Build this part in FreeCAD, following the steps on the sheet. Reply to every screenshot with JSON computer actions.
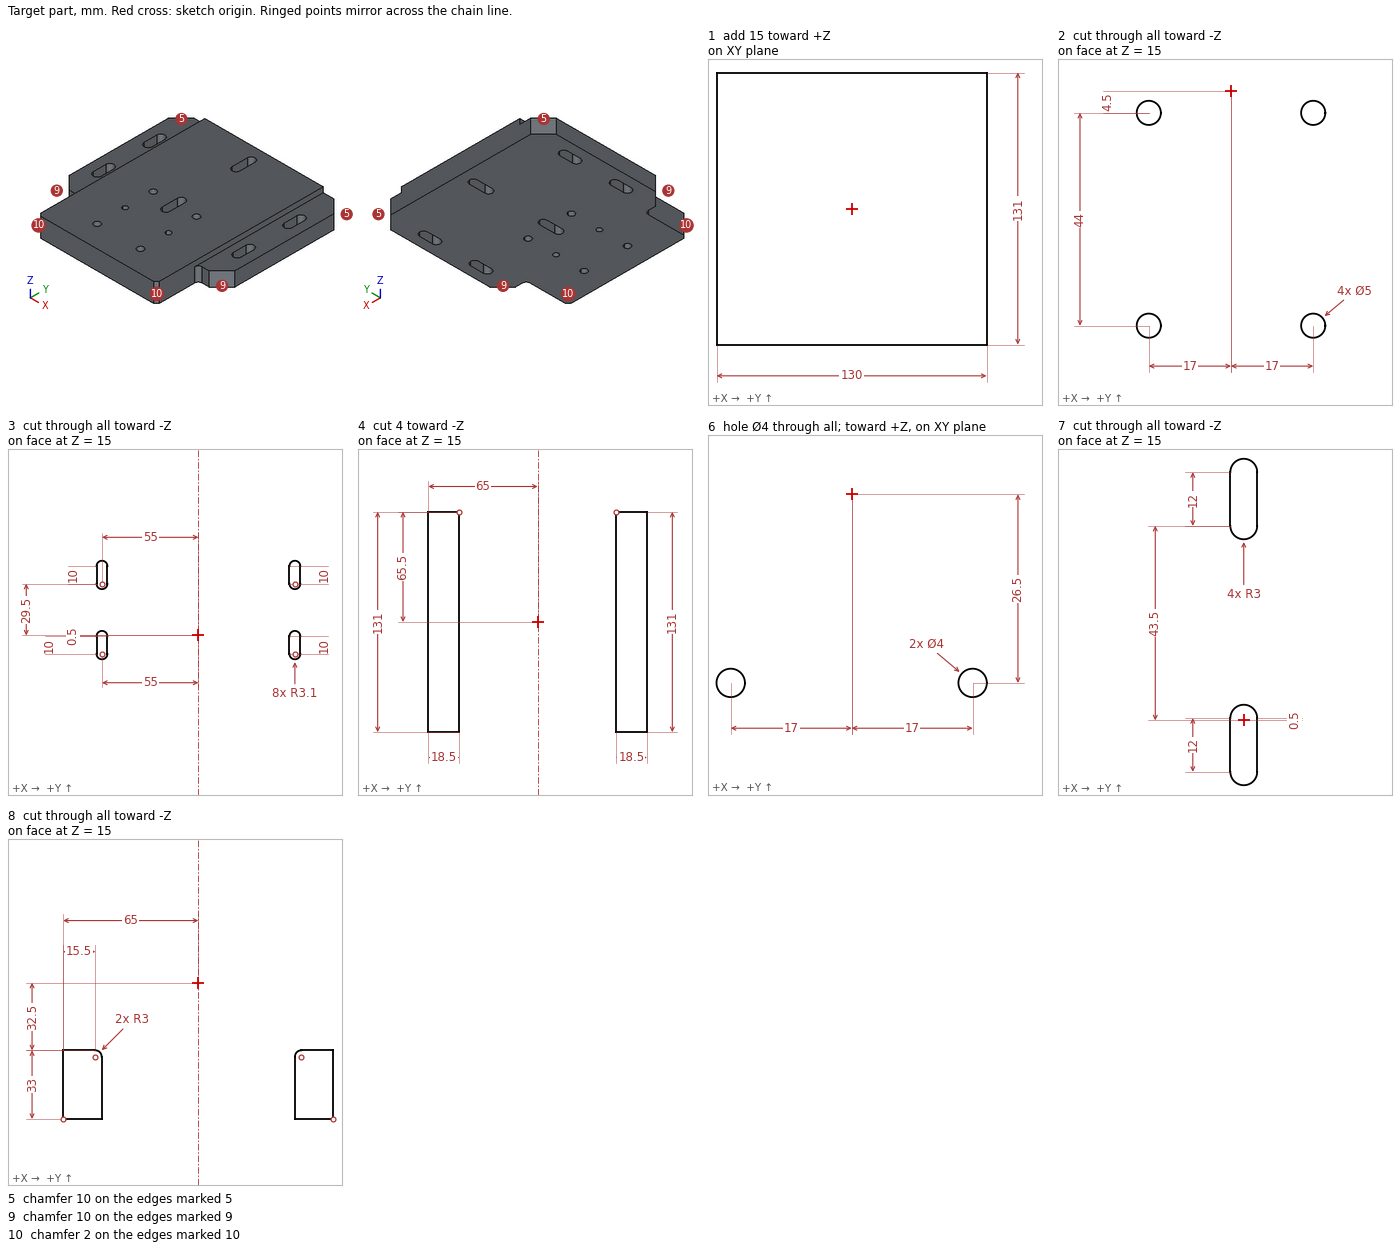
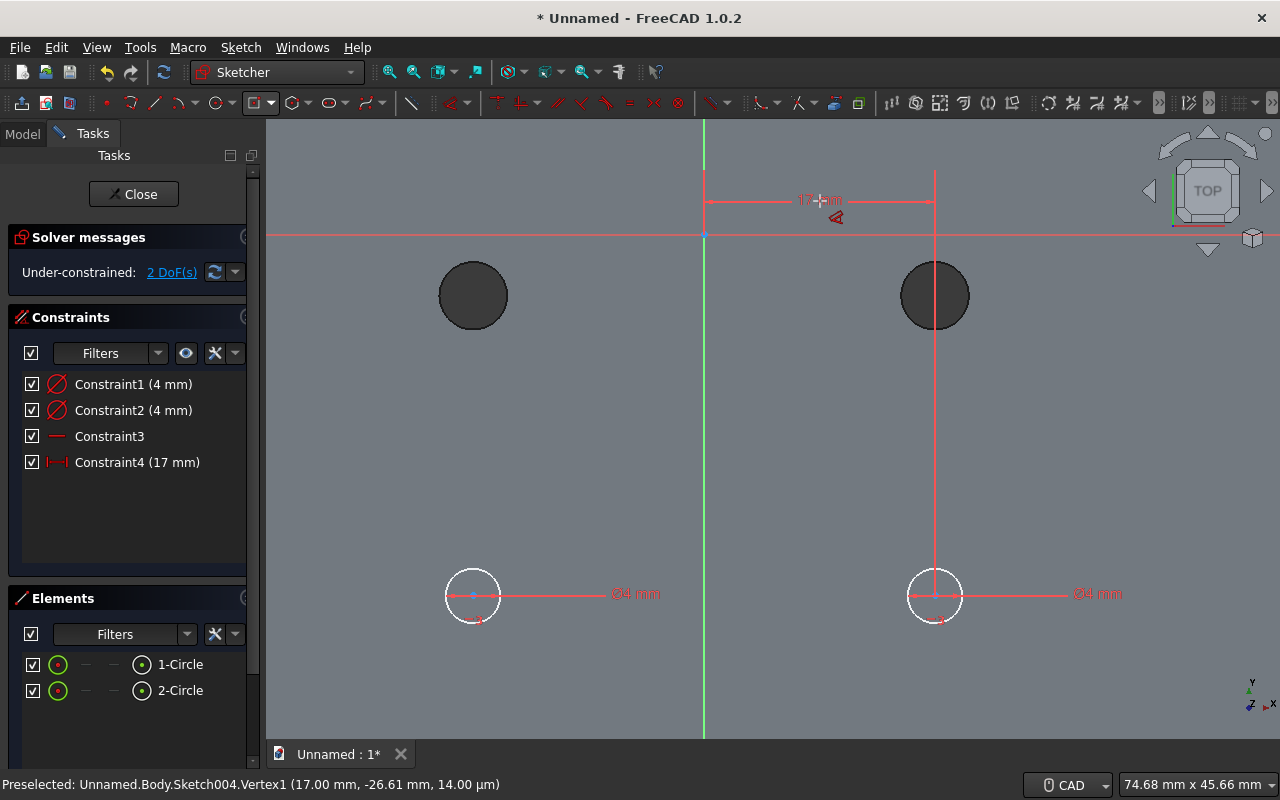
{"action": "left_click", "coordinate": [473, 596]}
{"action": "left_click", "coordinate": [589, 201]}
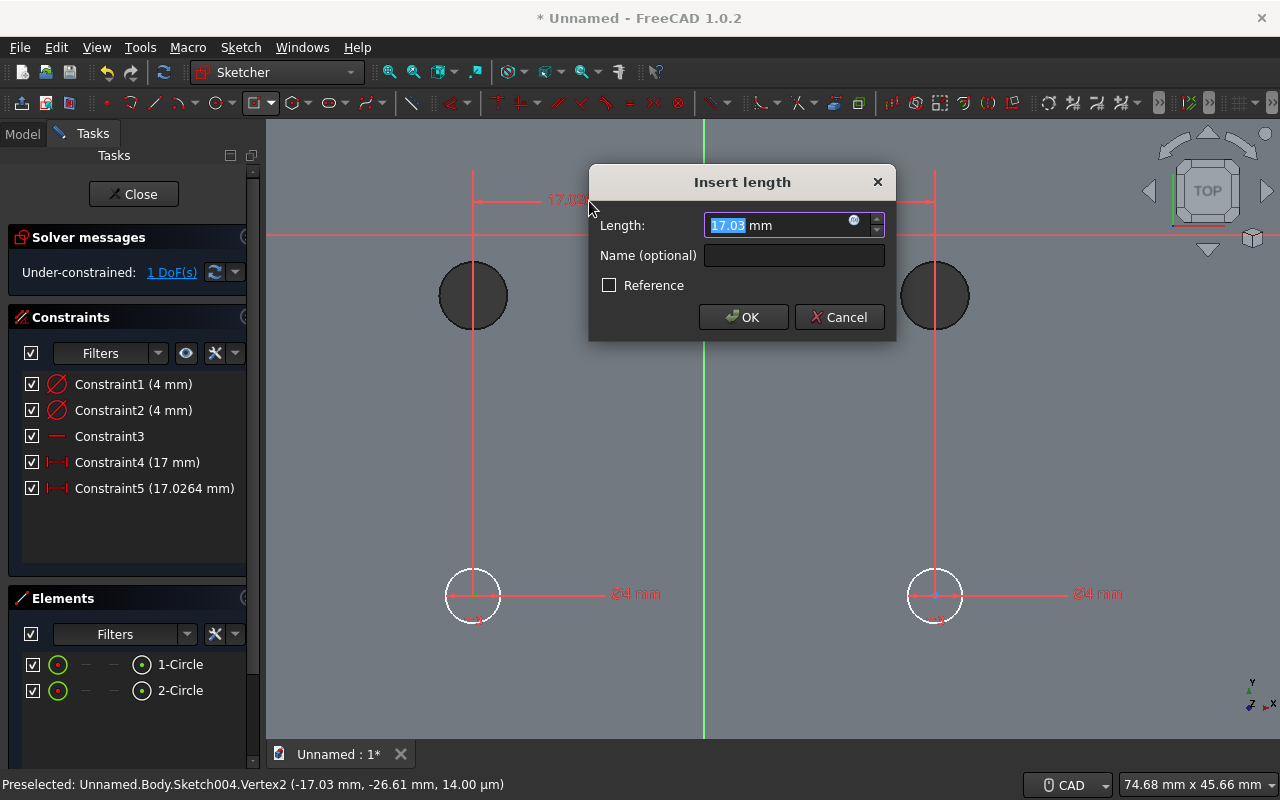
{"action": "type", "text": "17"}
{"action": "key", "text": "Return"}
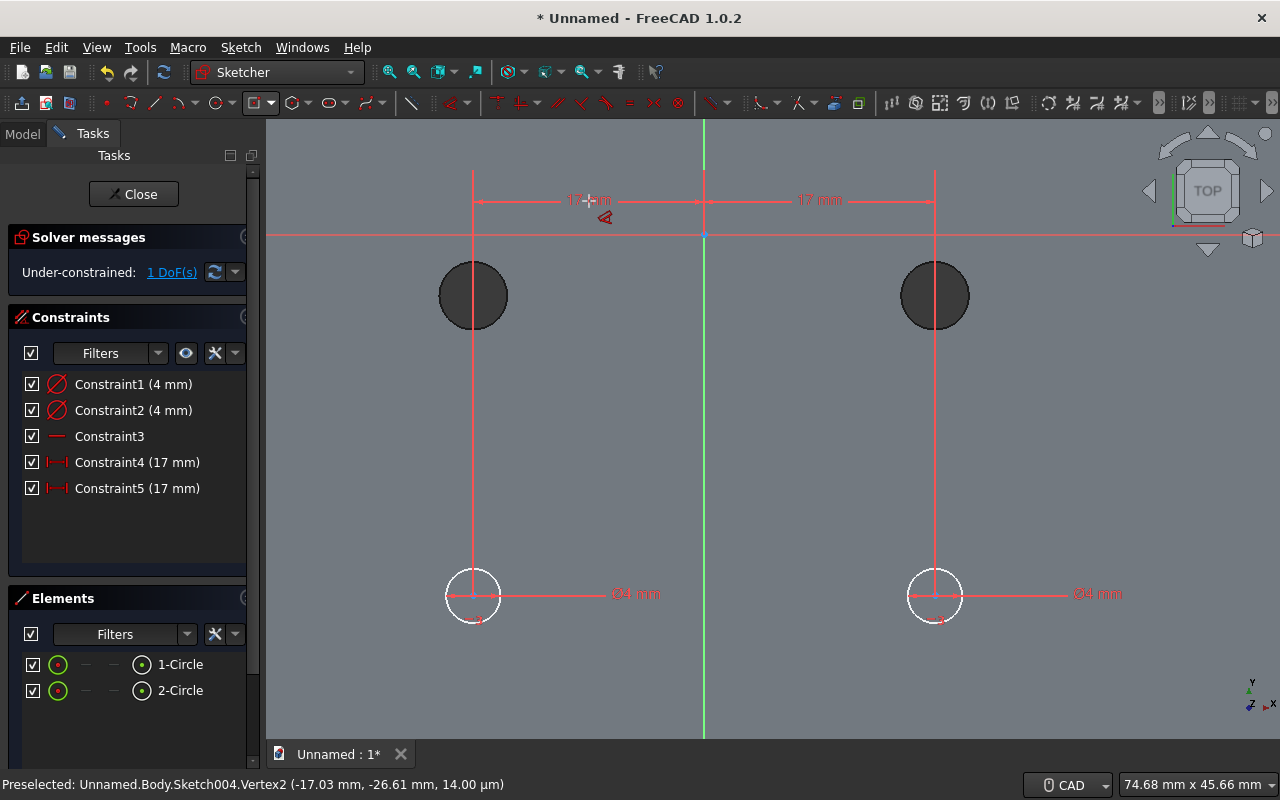
{"action": "left_click", "coordinate": [935, 596]}
{"action": "left_click", "coordinate": [969, 415]}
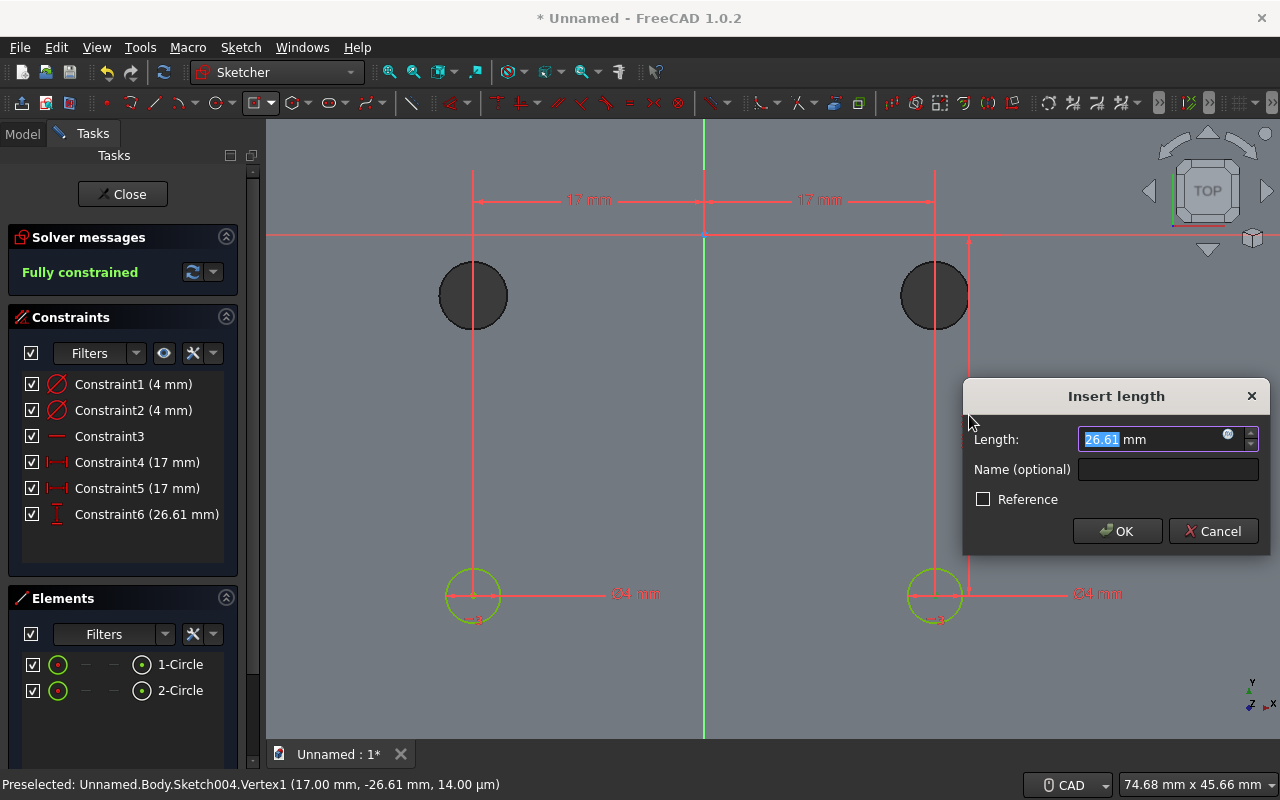
{"action": "type", "text": "26.5"}
{"action": "key", "text": "Return"}
{"action": "key", "text": "Escape"}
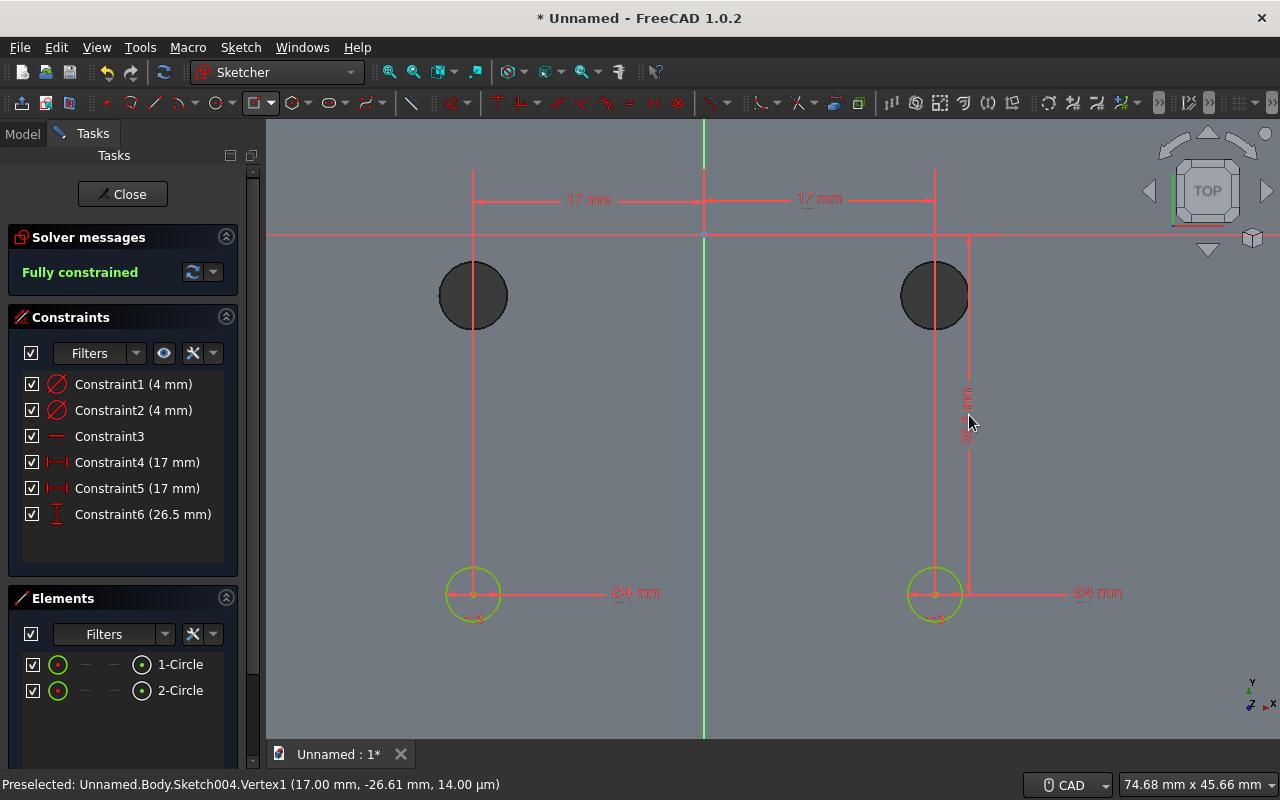
{"action": "left_click", "coordinate": [123, 194]}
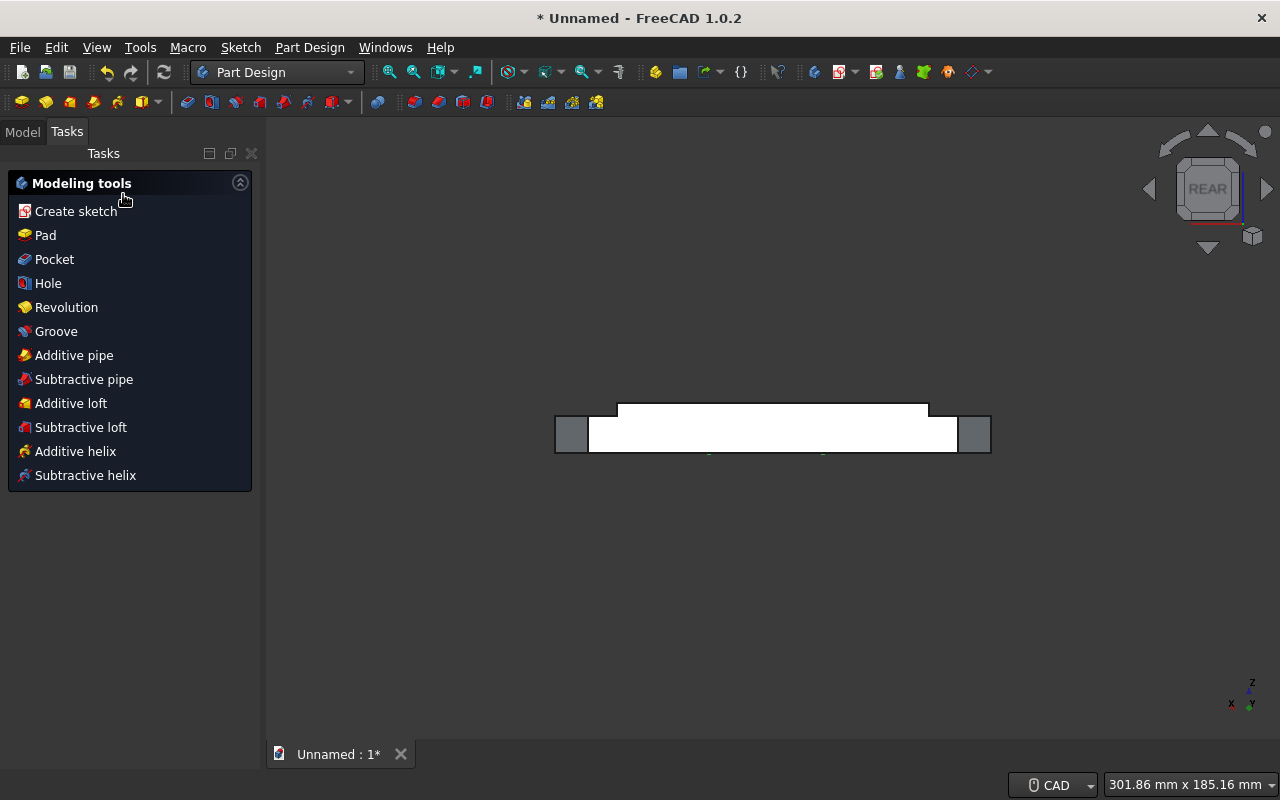
{"action": "left_click", "coordinate": [212, 102]}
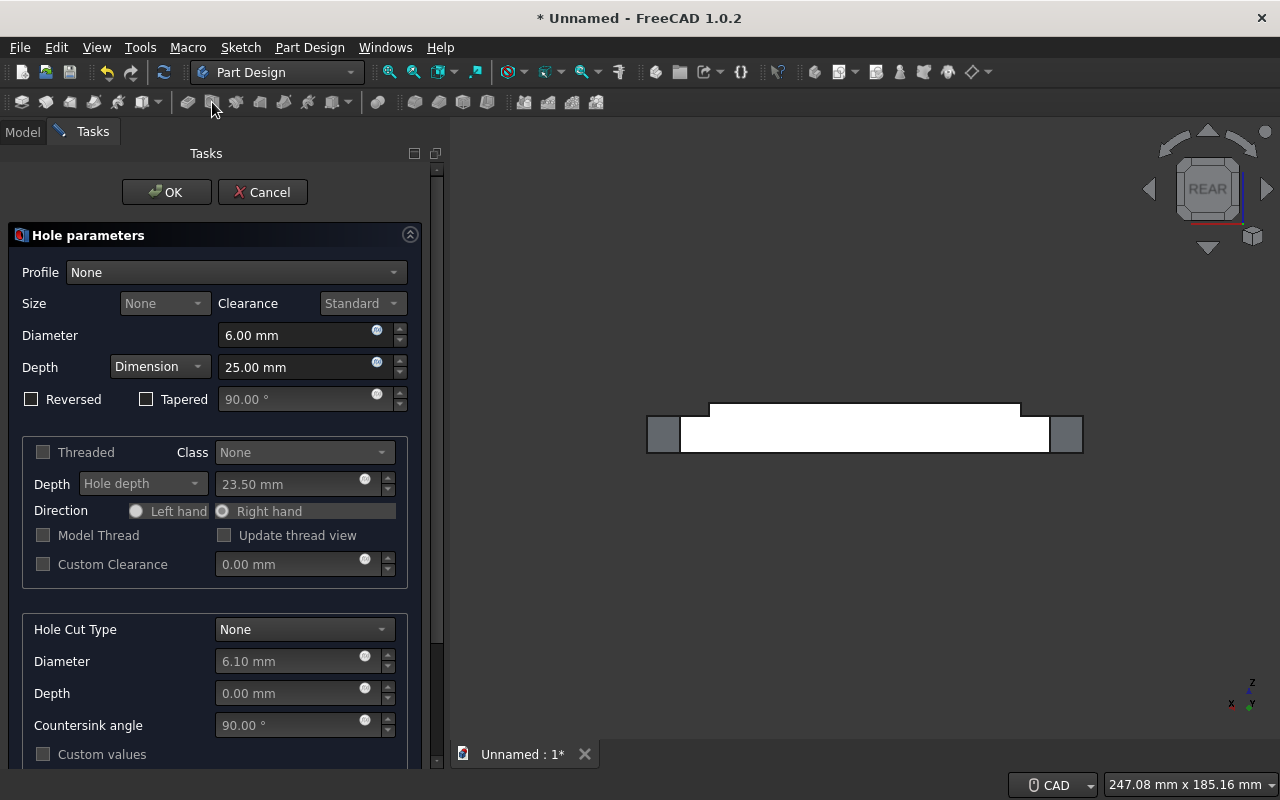
{"action": "triple_click", "coordinate": [305, 335]}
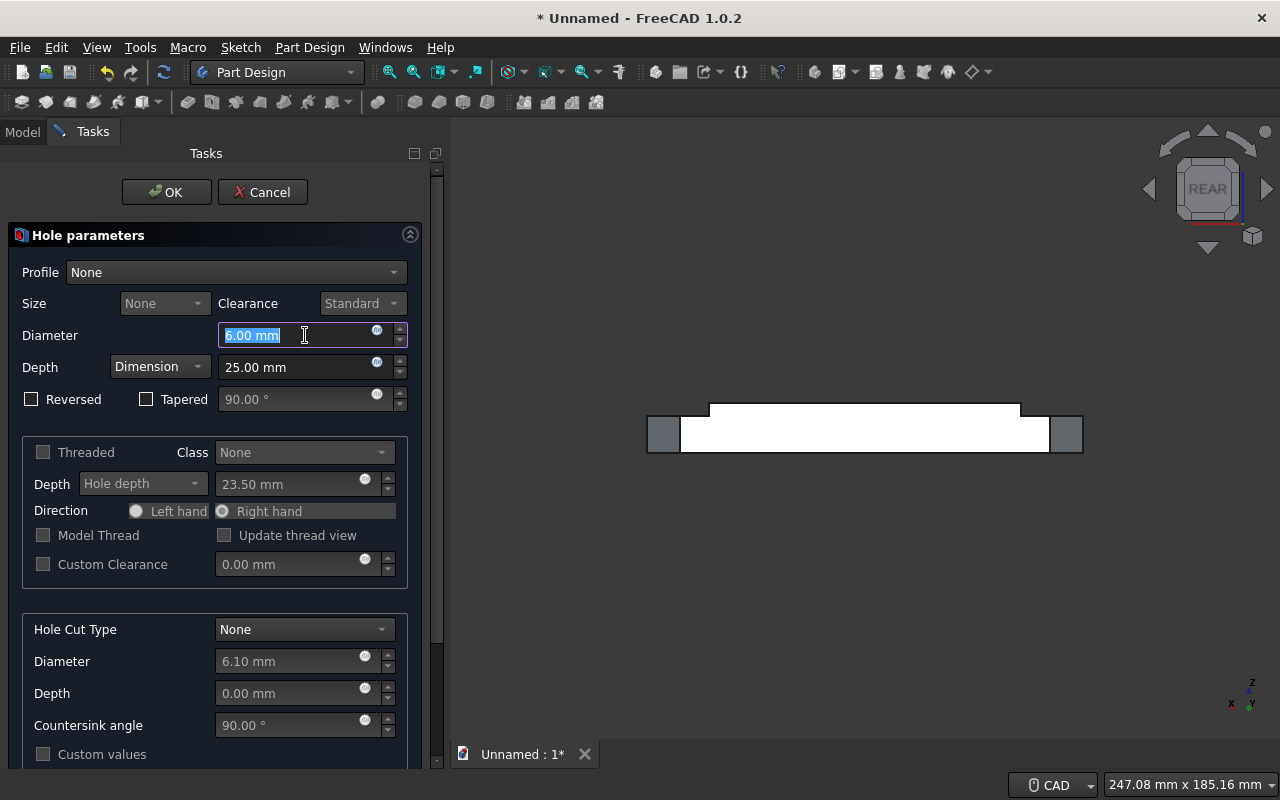
{"action": "type", "text": "4"}
{"action": "key", "text": "Tab"}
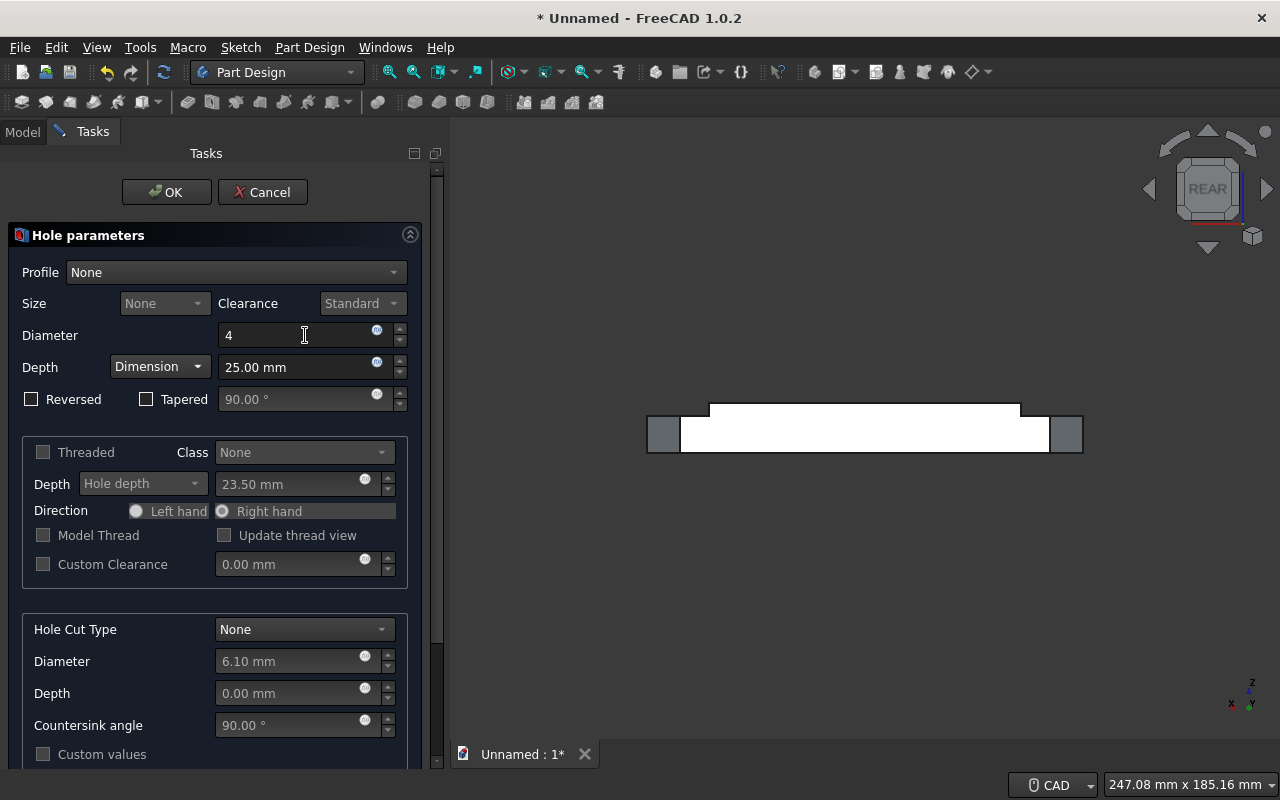
{"action": "left_click", "coordinate": [161, 366]}